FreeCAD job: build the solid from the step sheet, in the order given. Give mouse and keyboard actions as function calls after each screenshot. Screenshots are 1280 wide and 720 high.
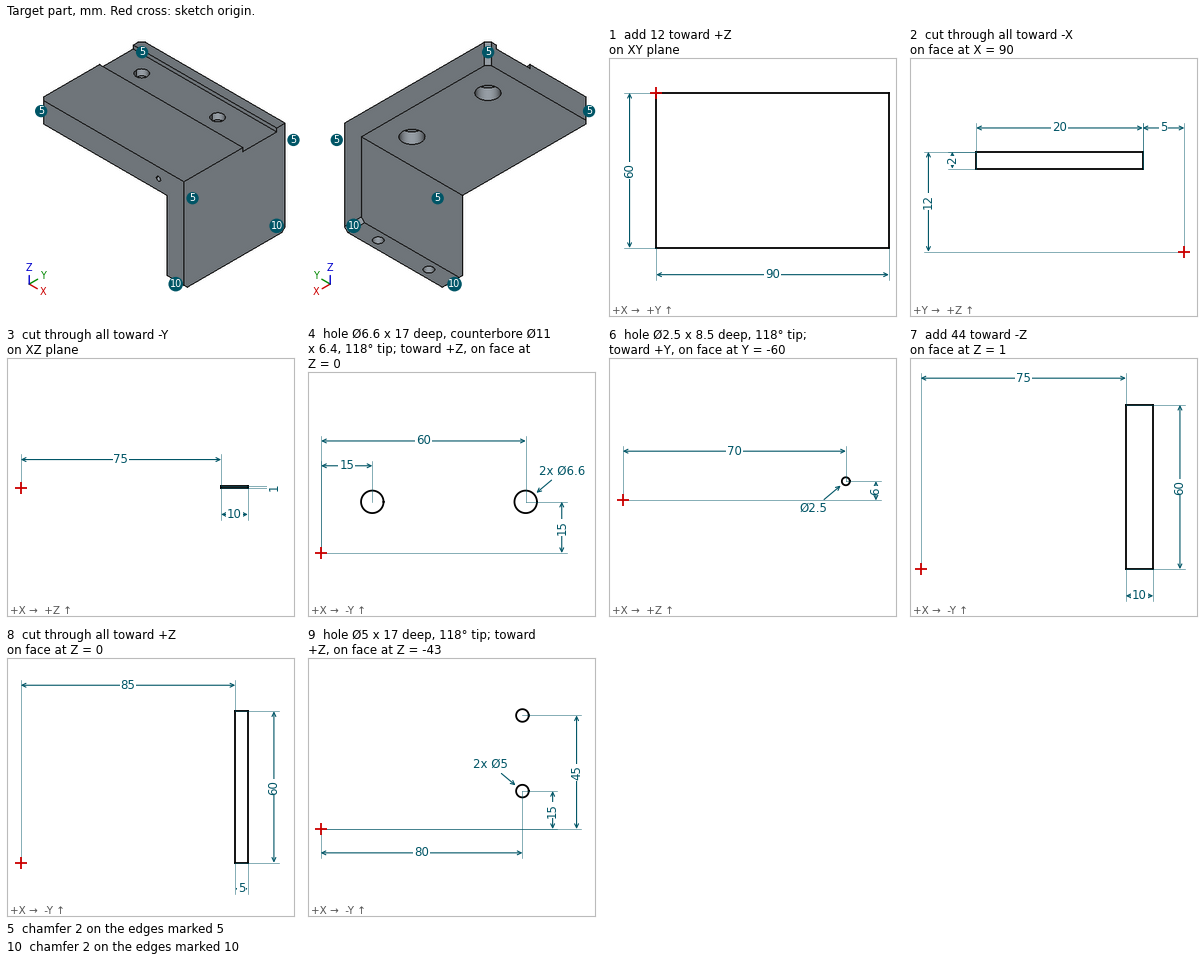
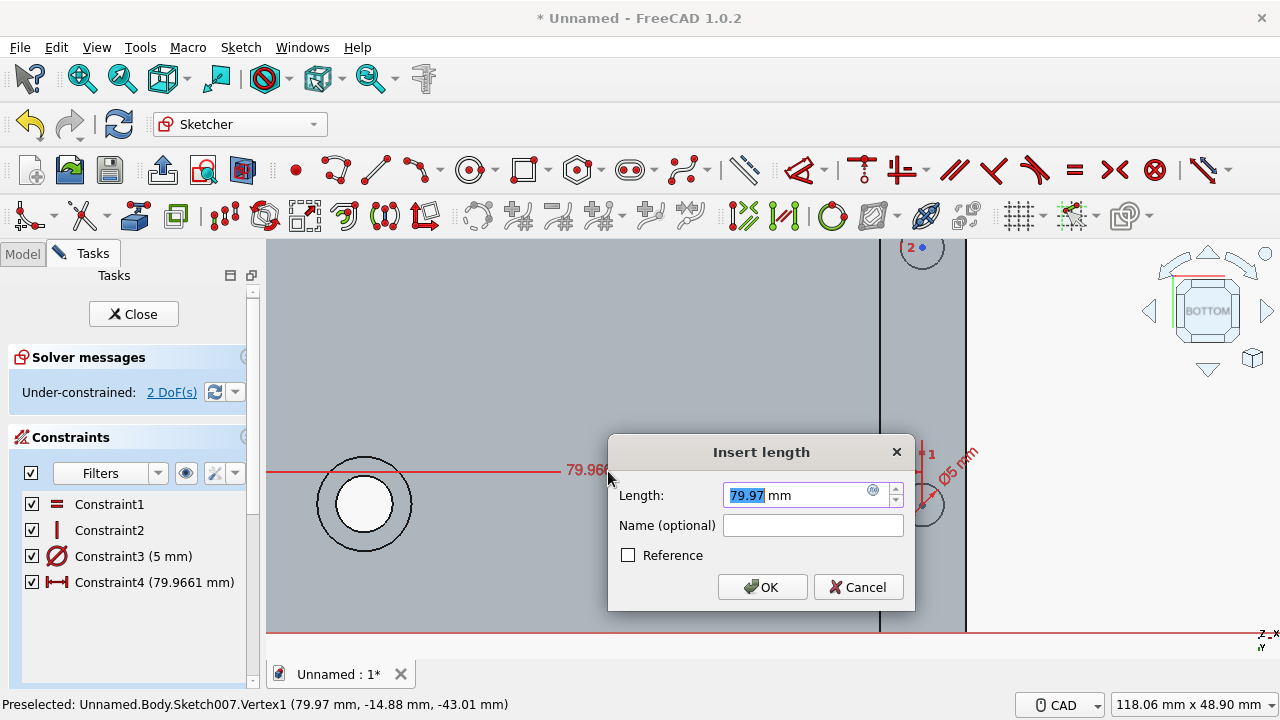
text(80)
key(Return)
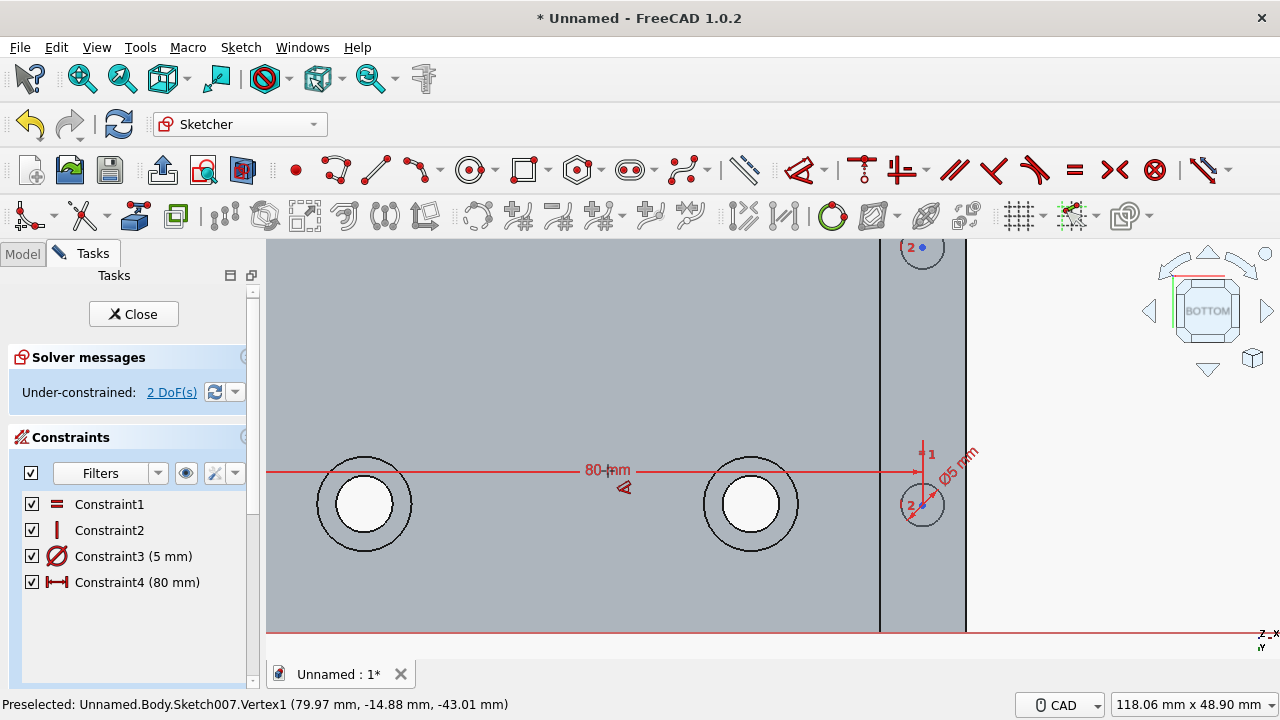
click(923, 505)
click(957, 568)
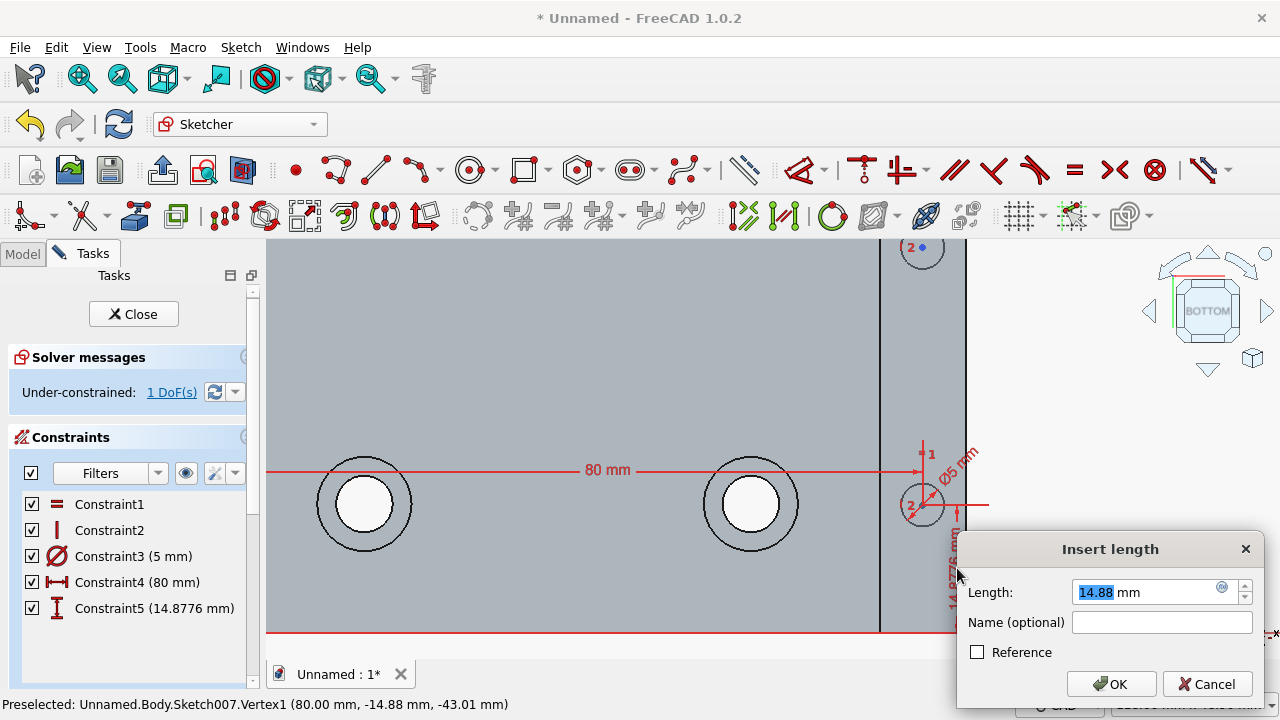
text(15)
key(Return)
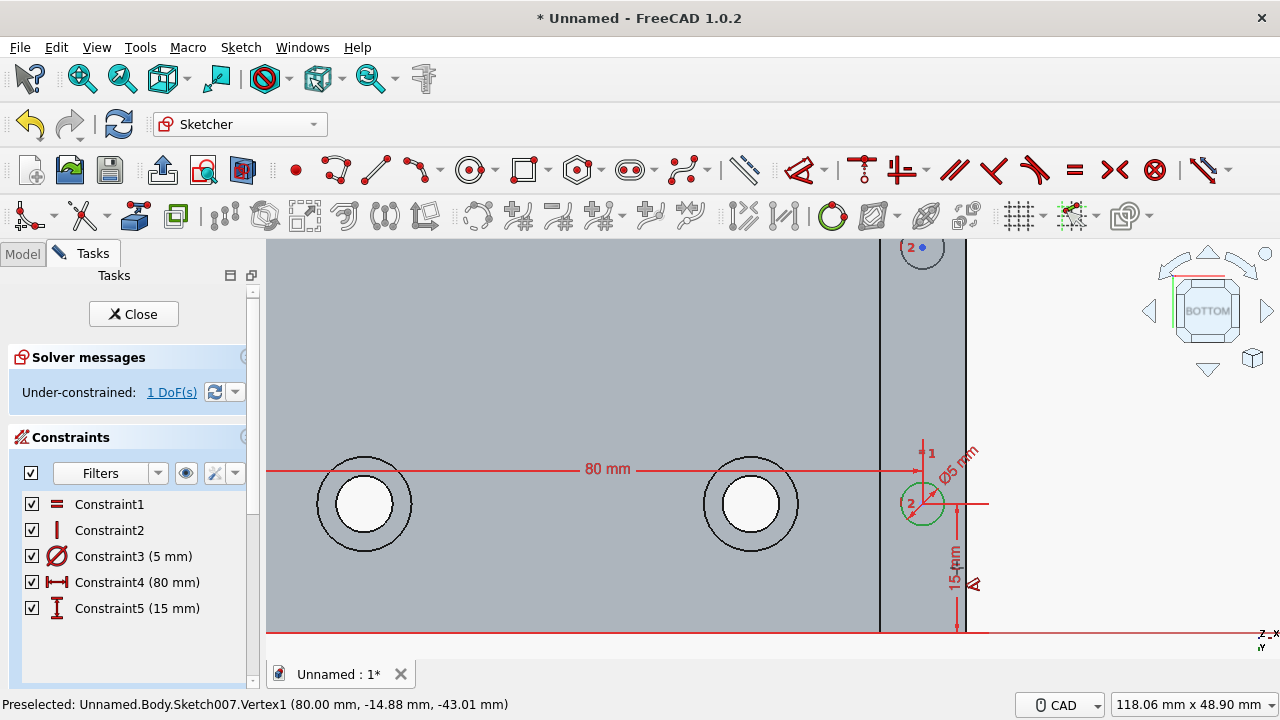
scroll(938, 490, down, 2)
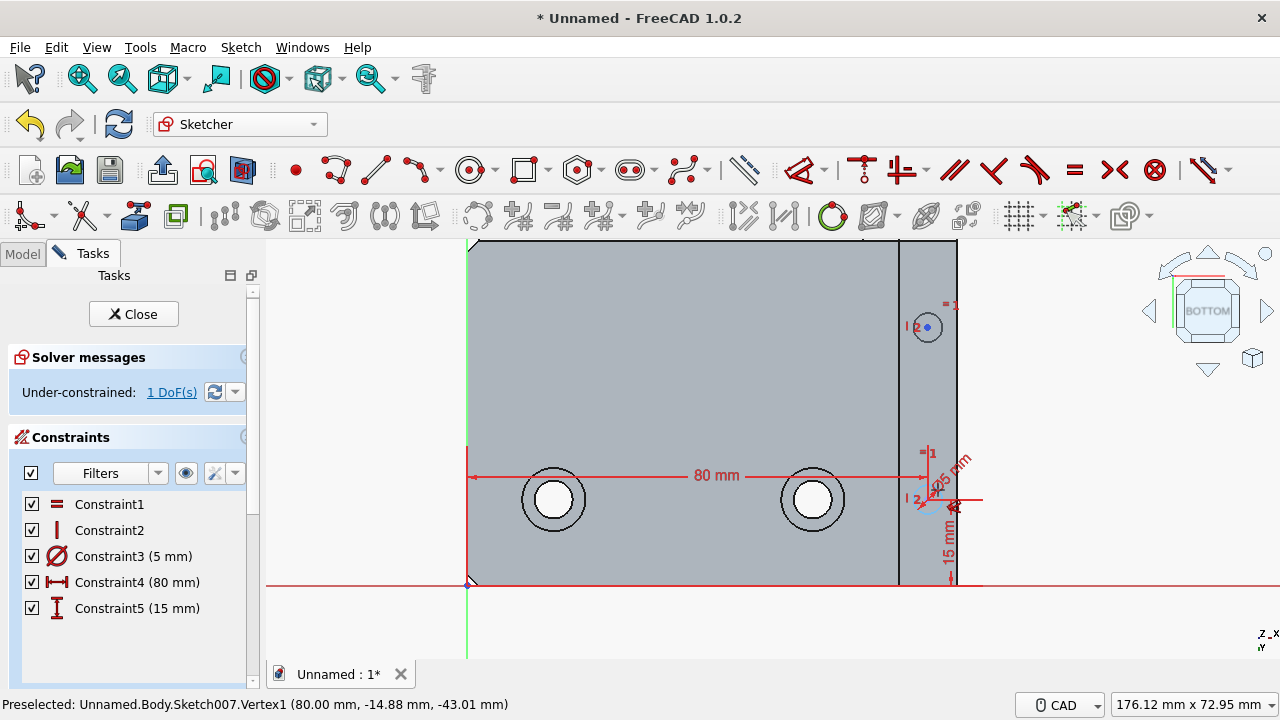
click(928, 328)
click(433, 457)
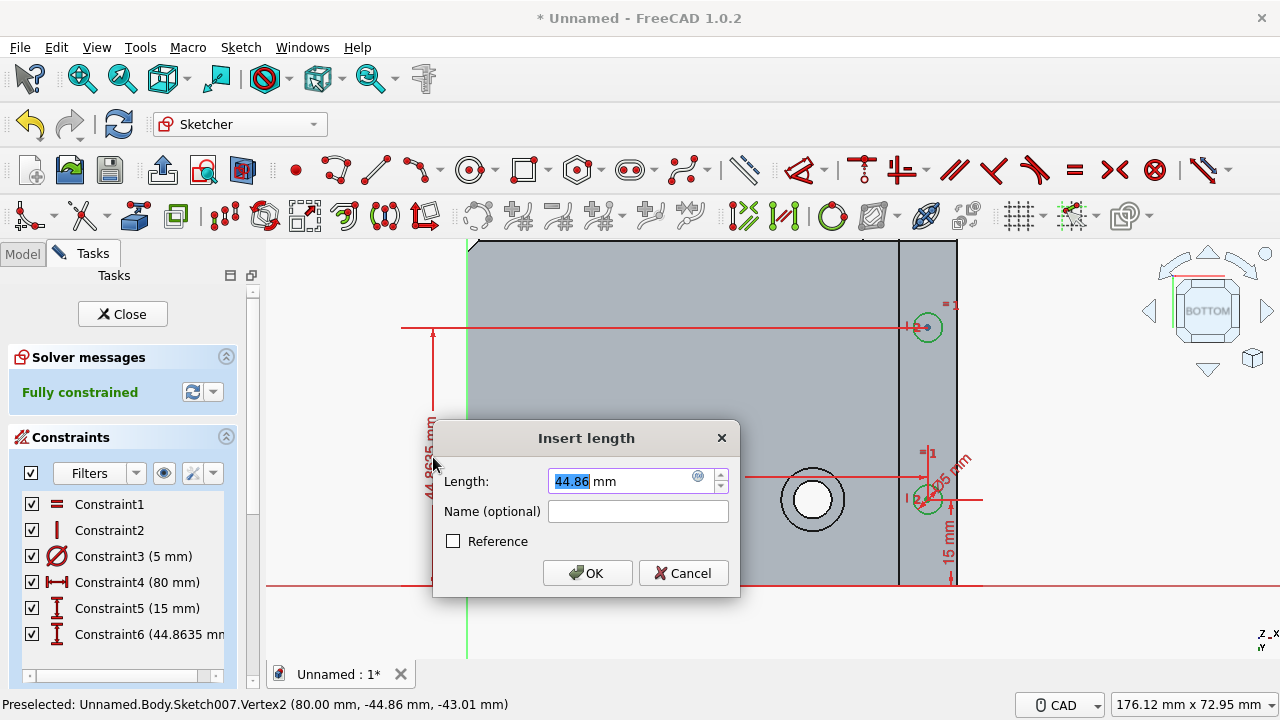
text(45)
key(Return)
key(Escape)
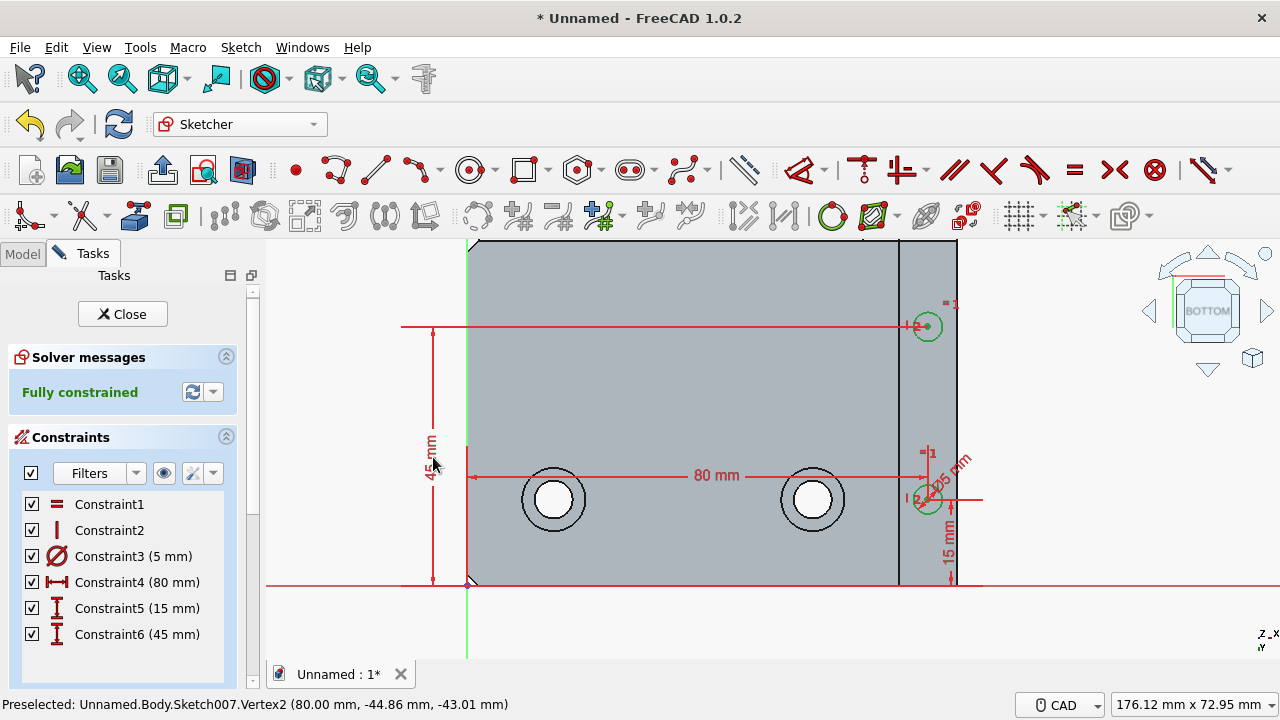
click(123, 314)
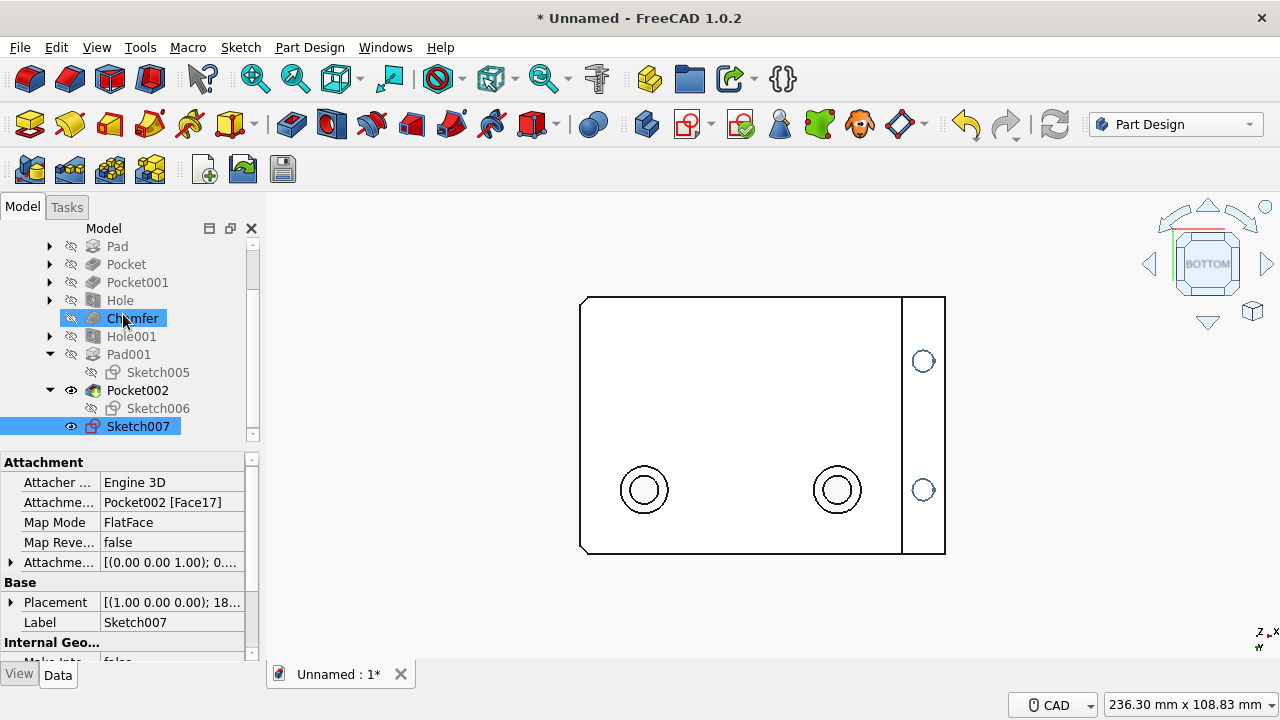
click(332, 124)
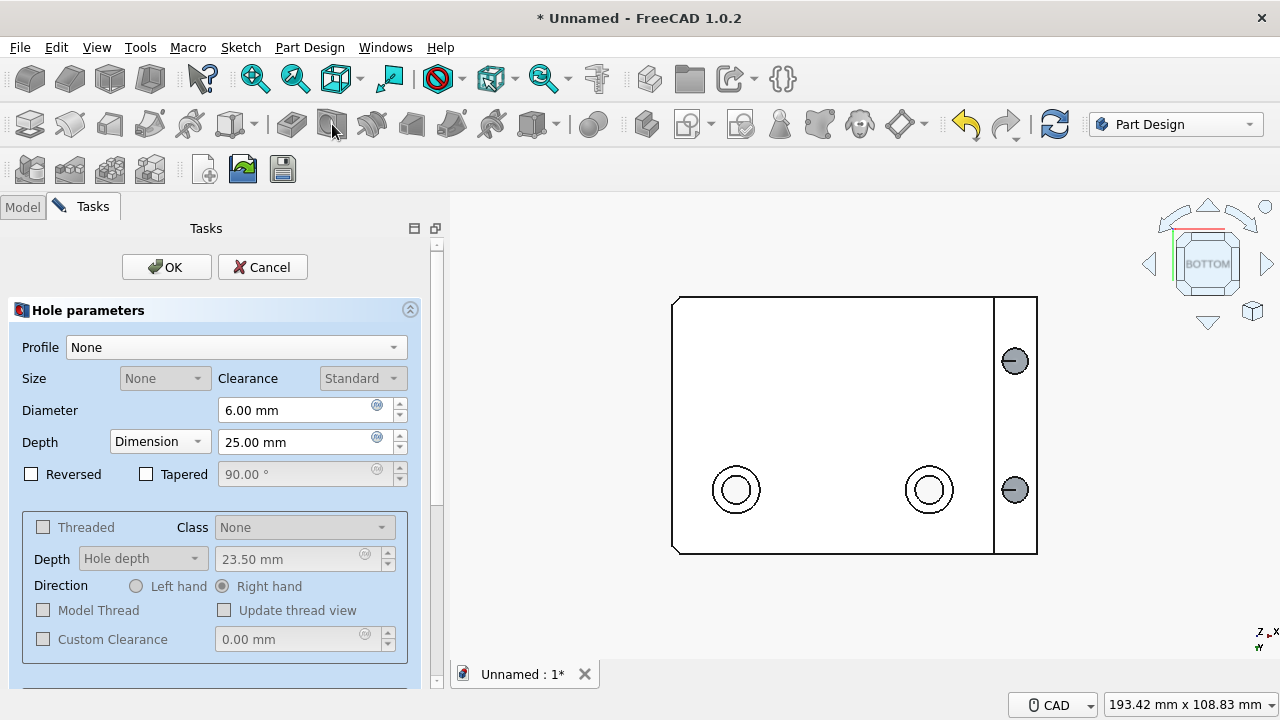
triple_click(305, 410)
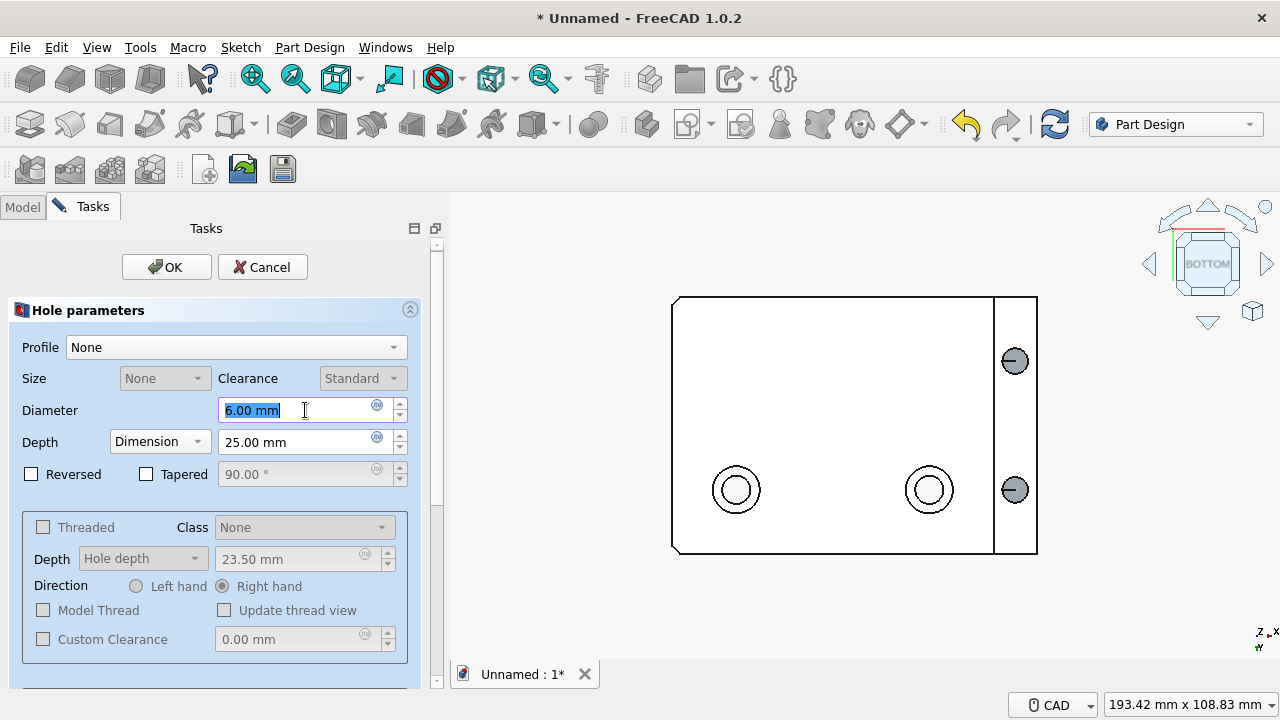
text(5)
key(Tab)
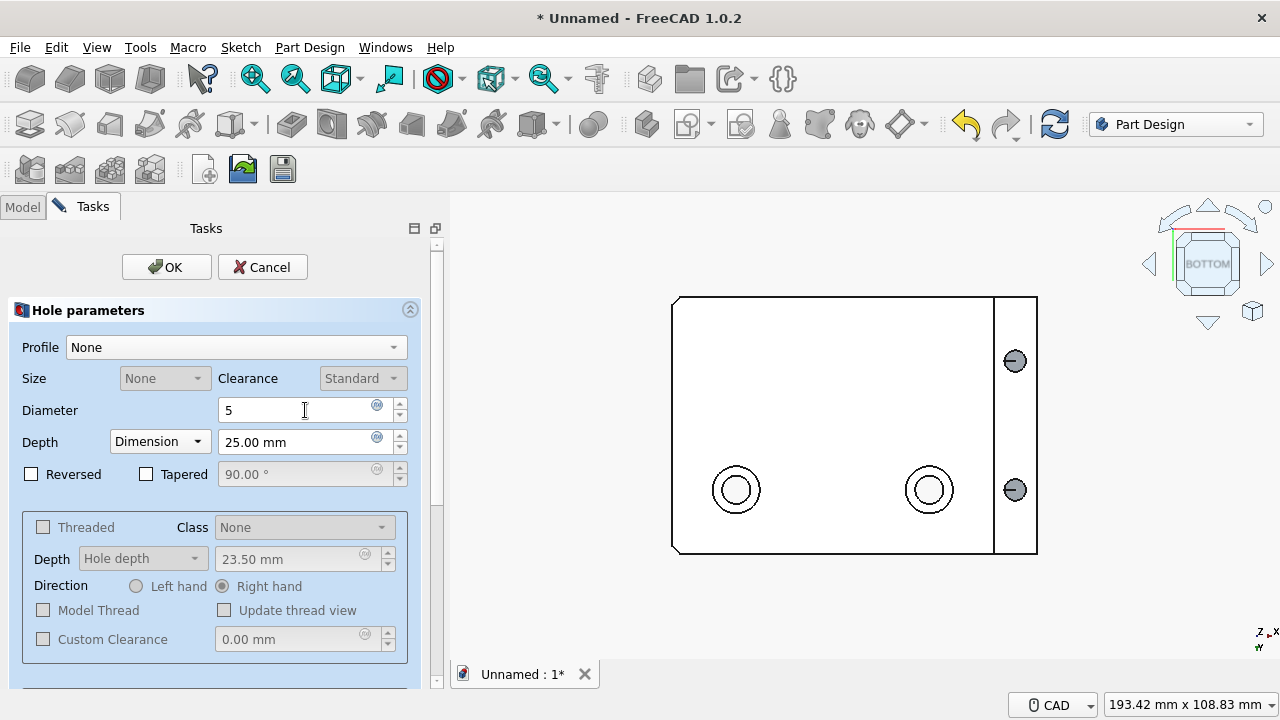
triple_click(305, 442)